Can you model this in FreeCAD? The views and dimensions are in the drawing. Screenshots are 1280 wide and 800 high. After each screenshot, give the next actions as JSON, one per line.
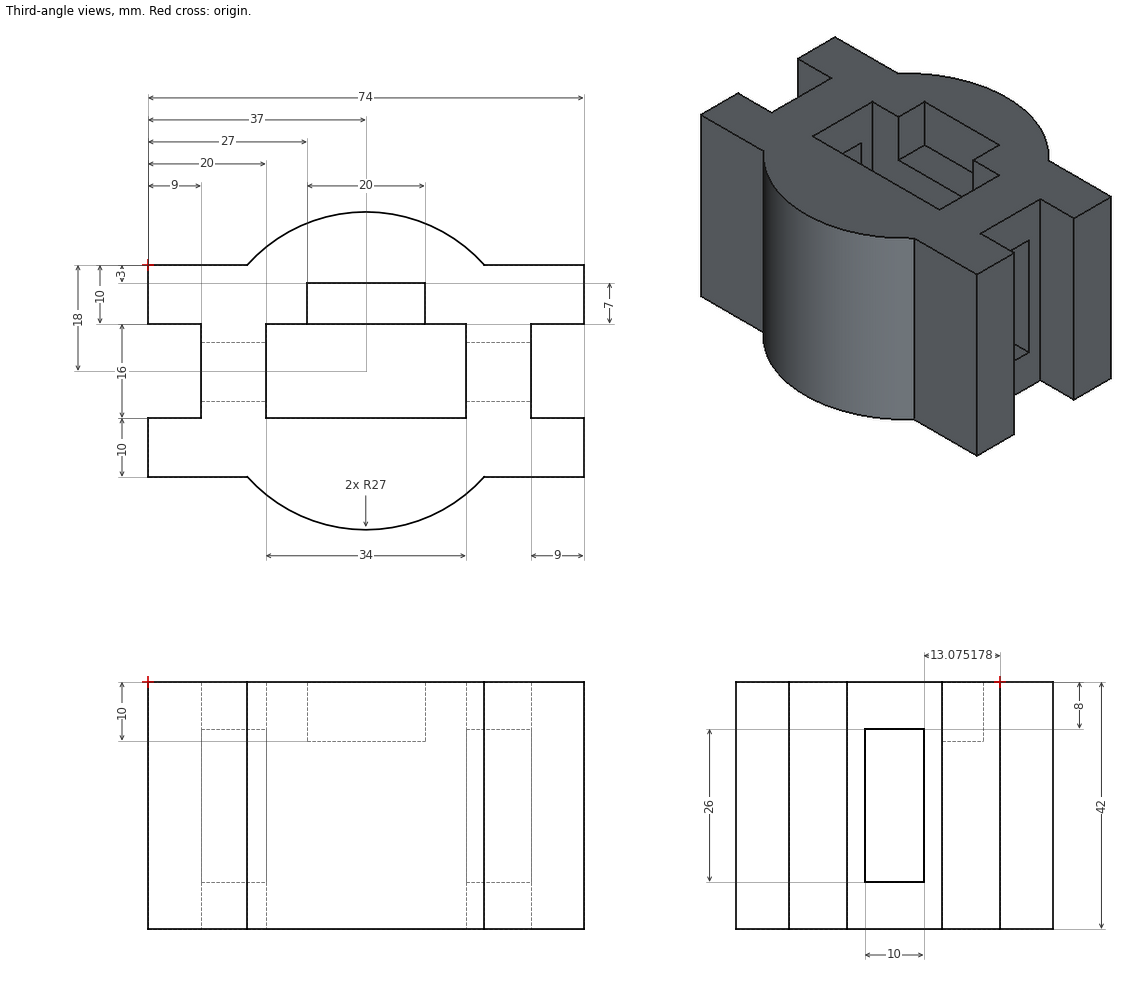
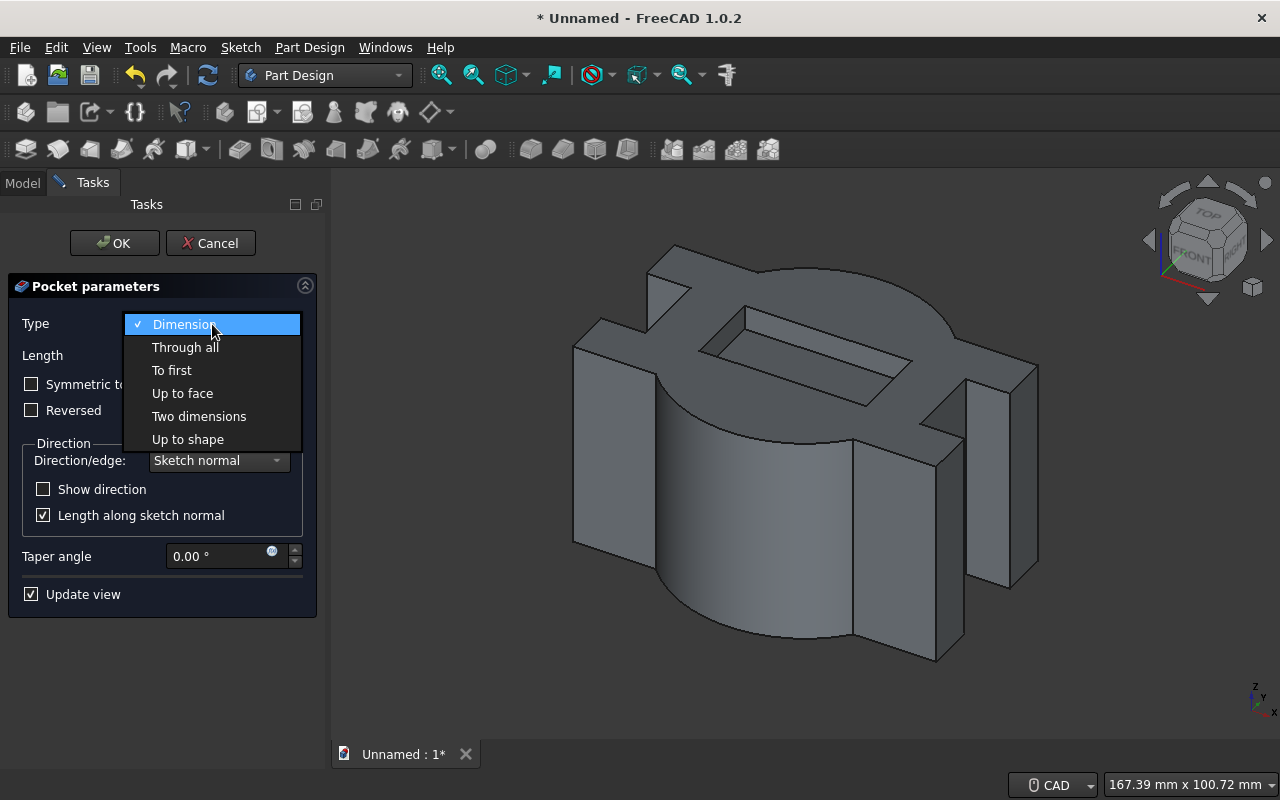
{"action": "left_click", "coordinate": [212, 348]}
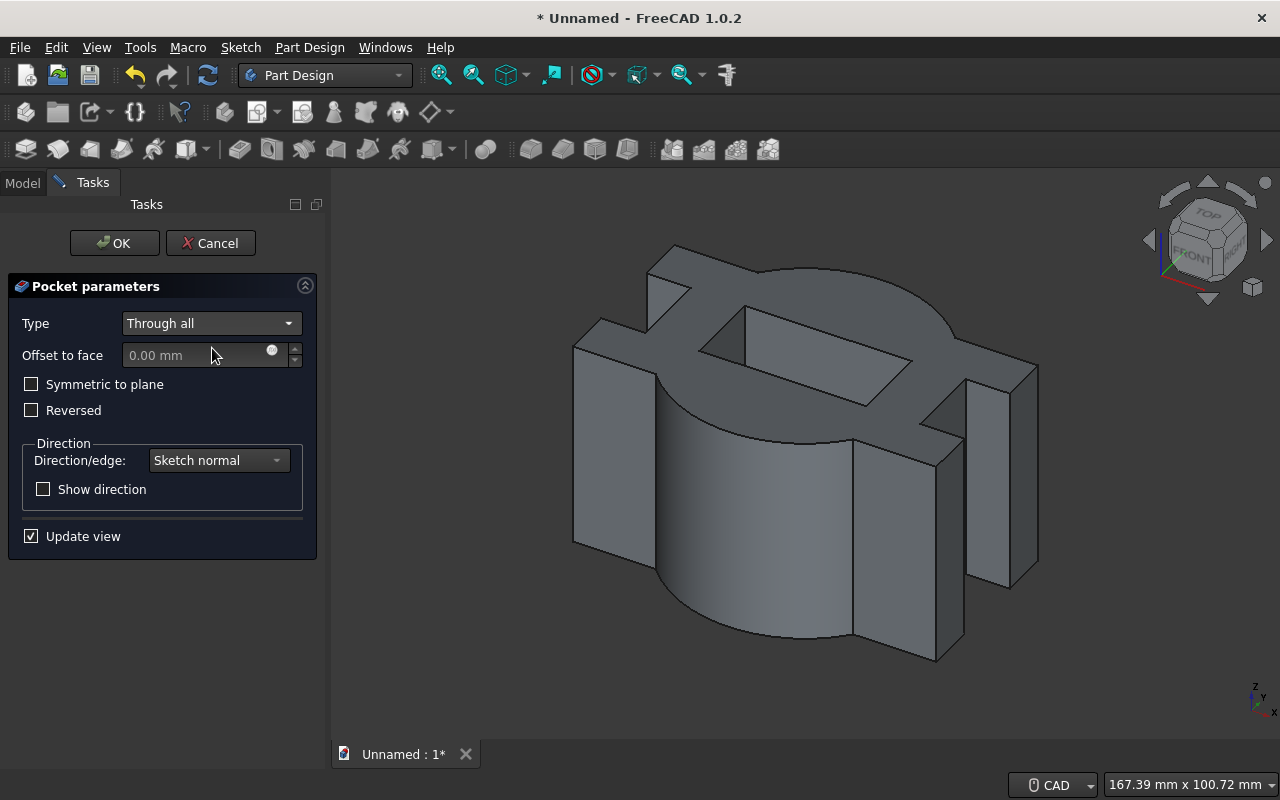
{"action": "left_click", "coordinate": [115, 243]}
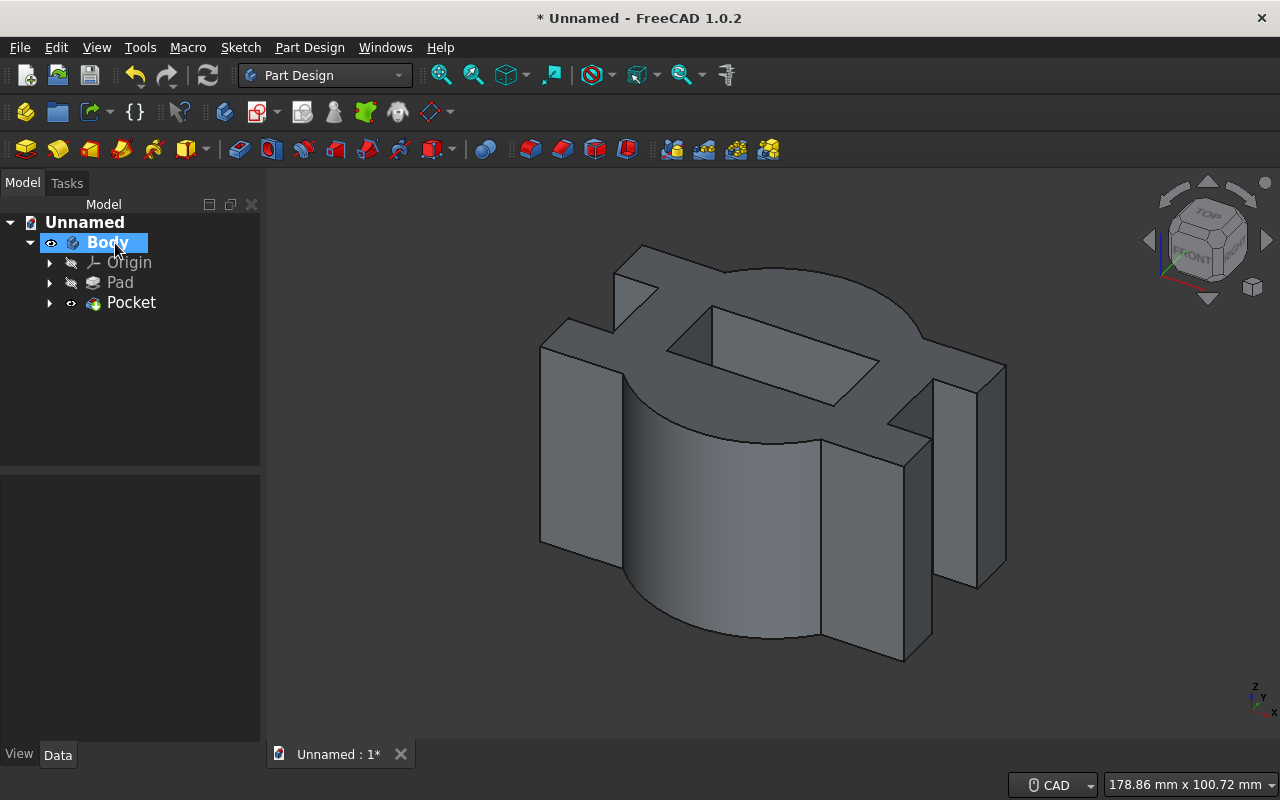
{"action": "left_click", "coordinate": [869, 329]}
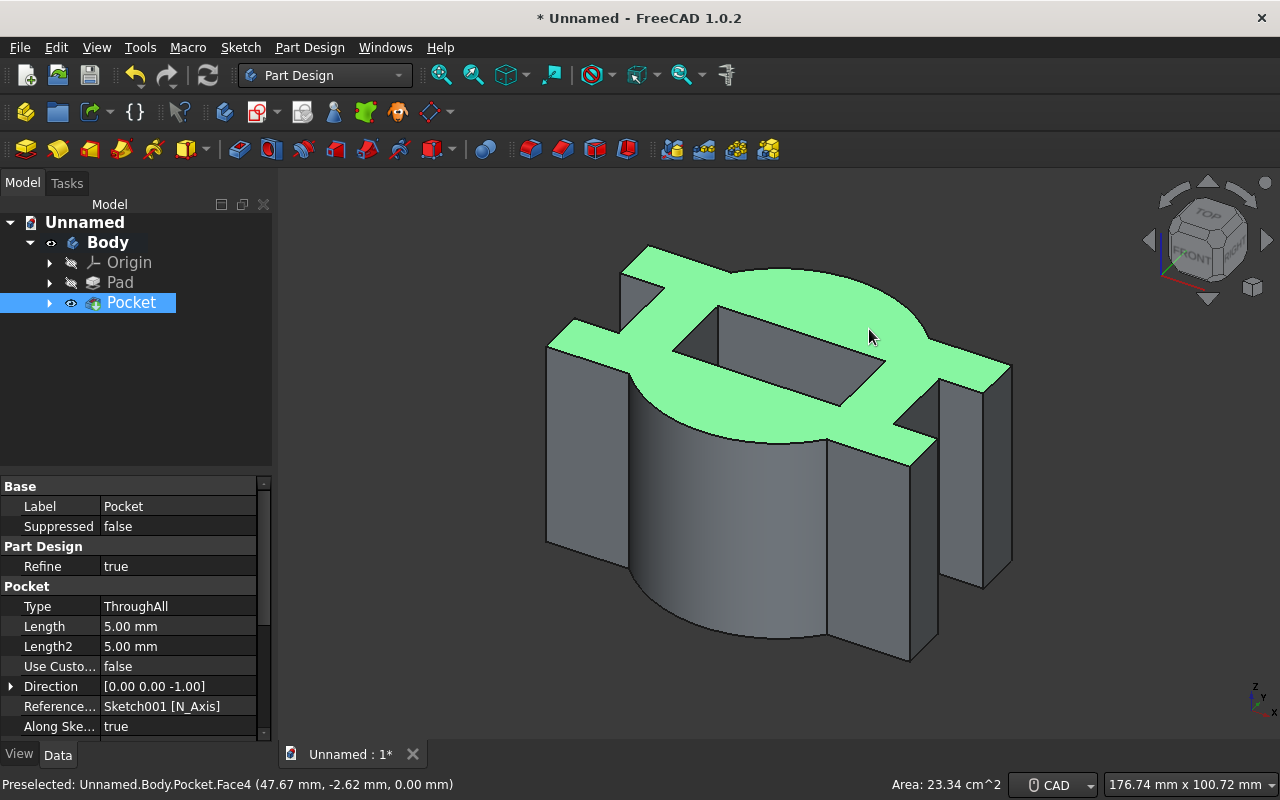
{"action": "left_click", "coordinate": [258, 112]}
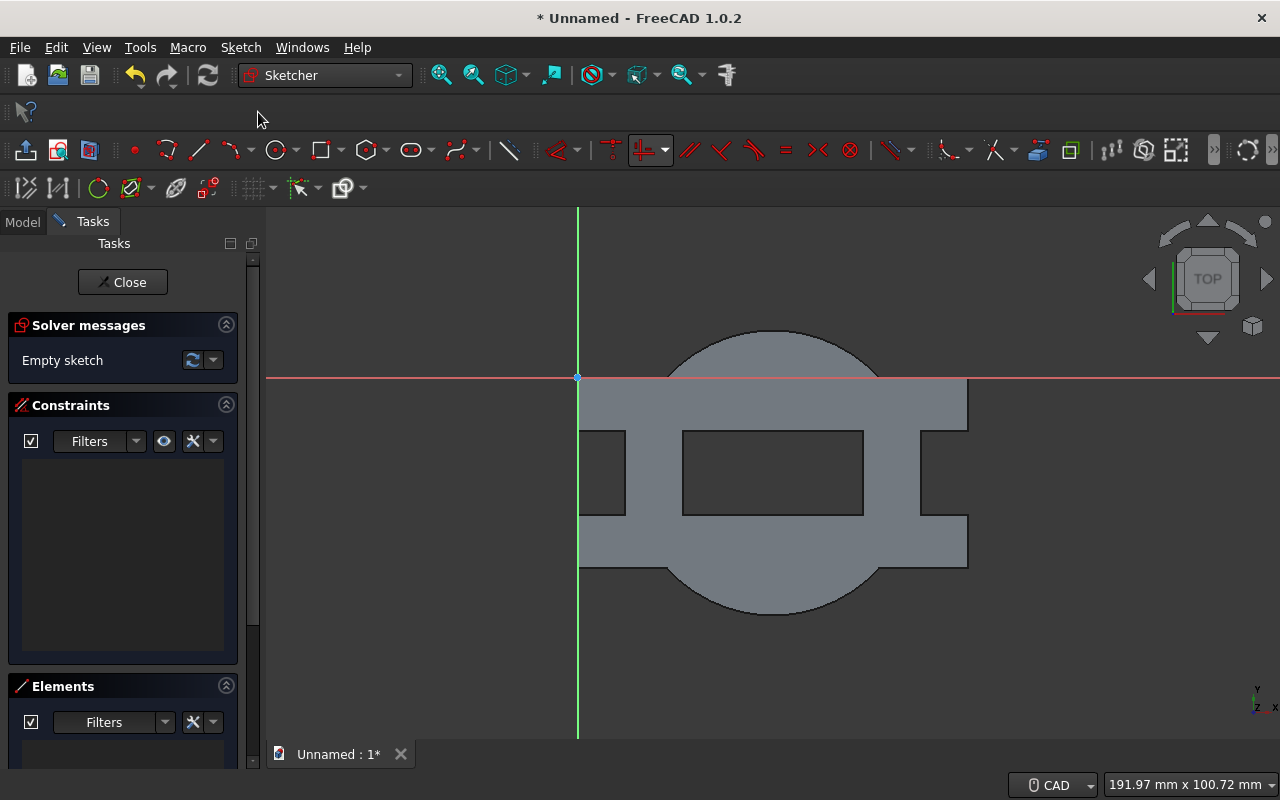
{"action": "scroll", "coordinate": [699, 348], "scroll_direction": "up", "scroll_amount": 4}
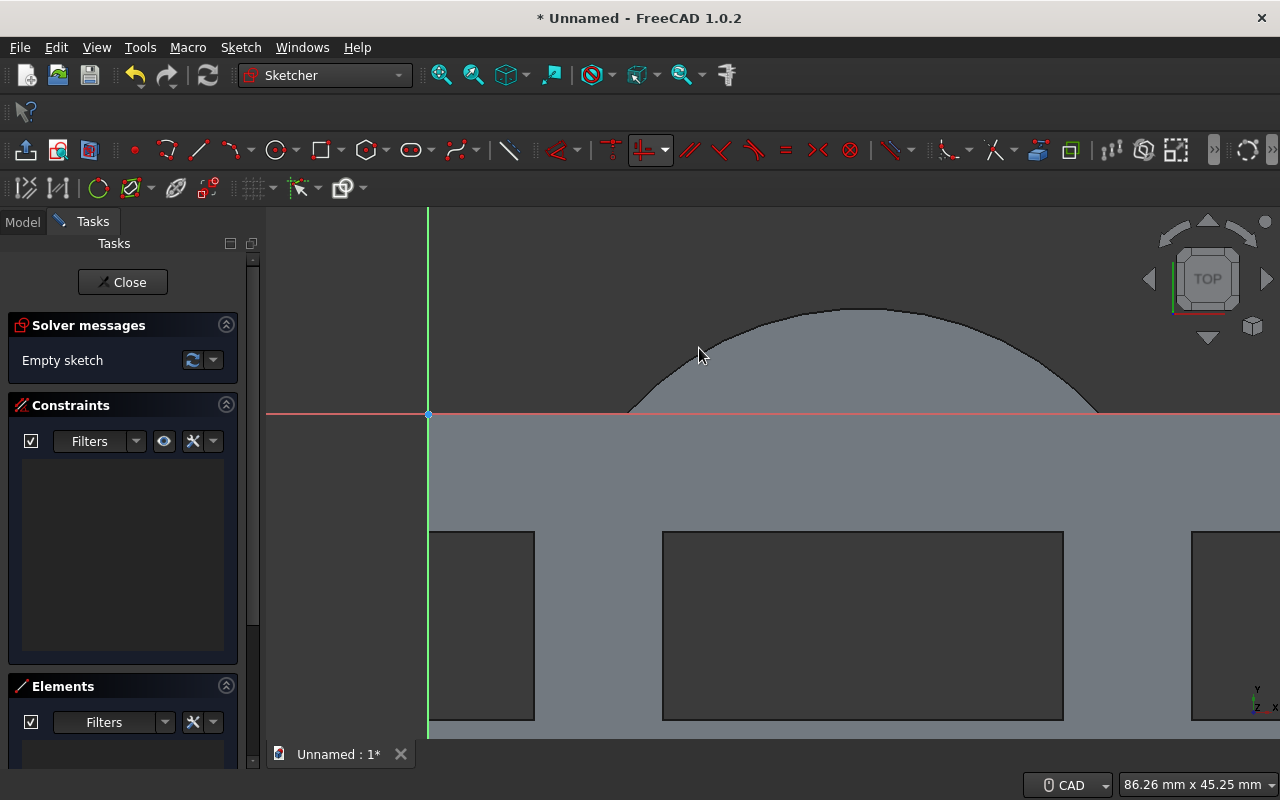
{"action": "left_click", "coordinate": [322, 150]}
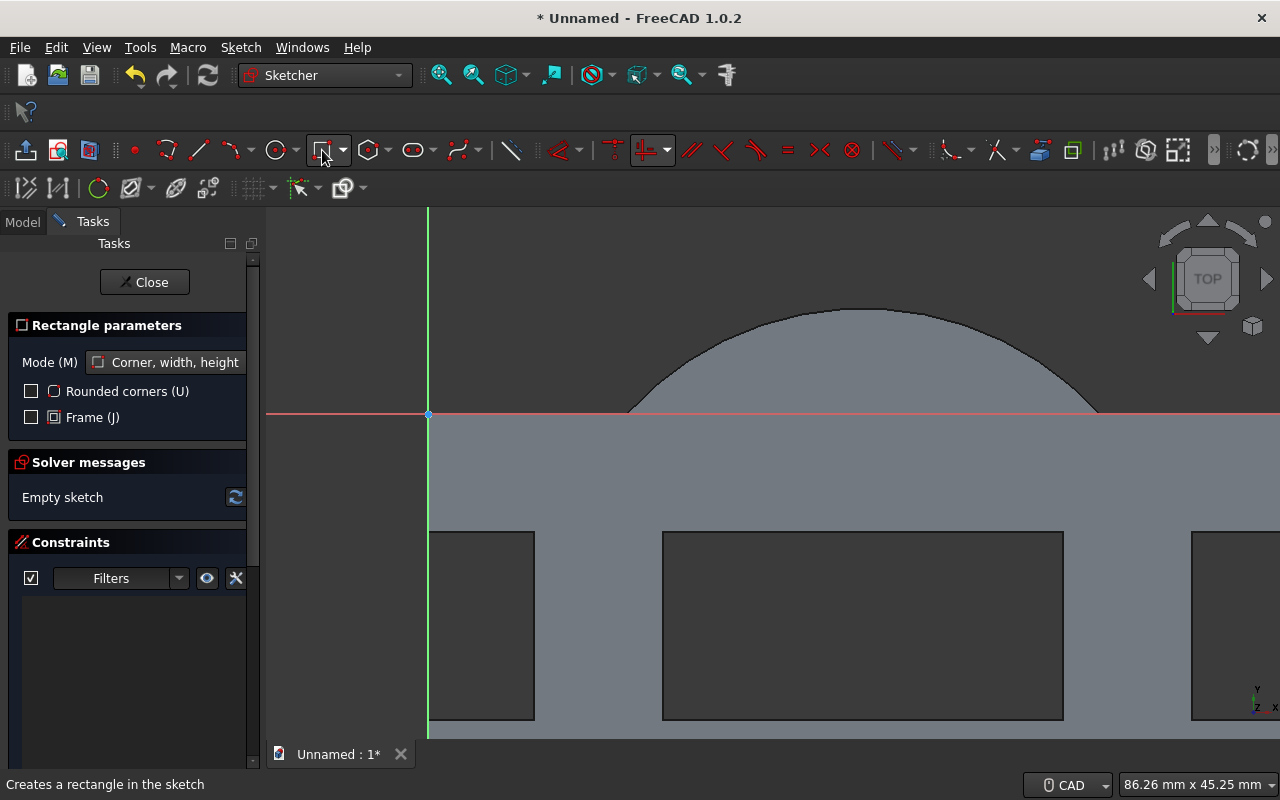
{"action": "left_click", "coordinate": [746, 450]}
{"action": "mouse_move", "coordinate": [981, 532]}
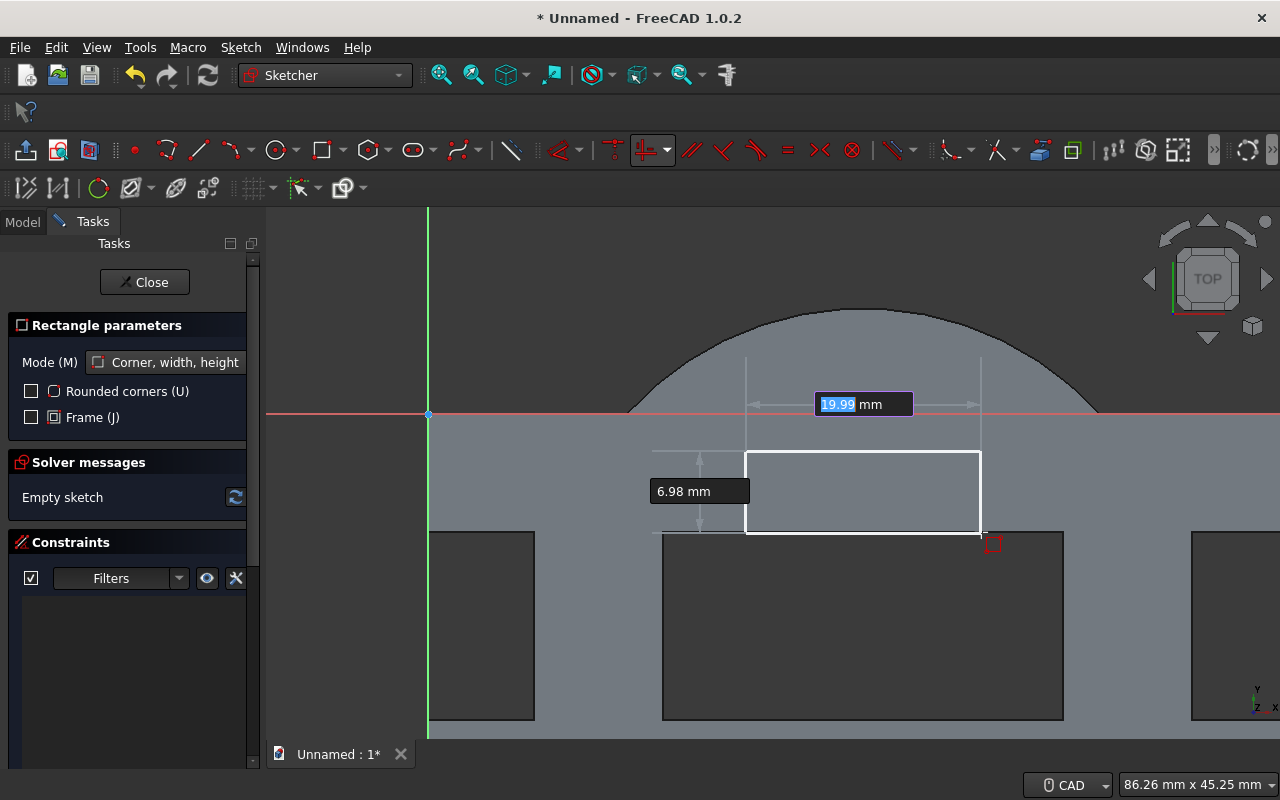
{"action": "type", "text": "20"}
{"action": "key", "text": "Tab"}
{"action": "type", "text": "7"}
{"action": "key", "text": "Return"}
{"action": "key", "text": "Escape"}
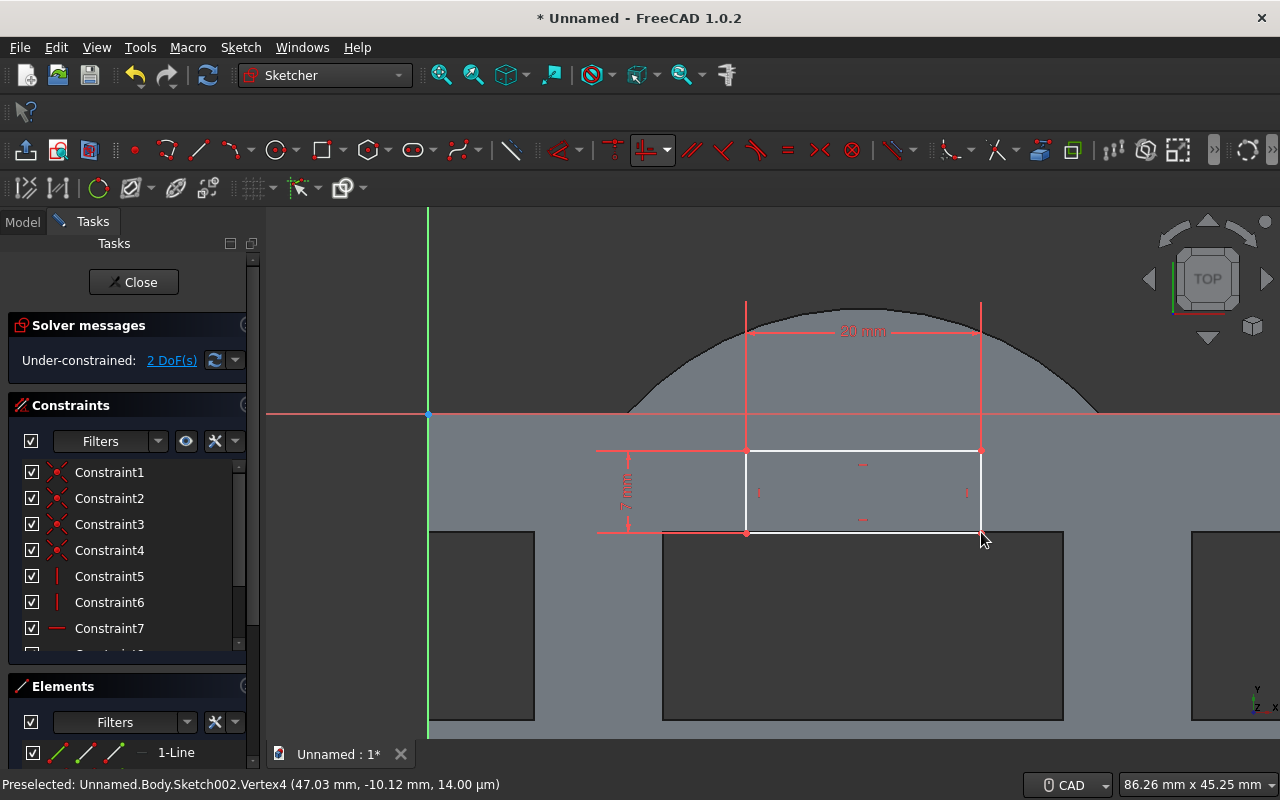
{"action": "left_click", "coordinate": [558, 150]}